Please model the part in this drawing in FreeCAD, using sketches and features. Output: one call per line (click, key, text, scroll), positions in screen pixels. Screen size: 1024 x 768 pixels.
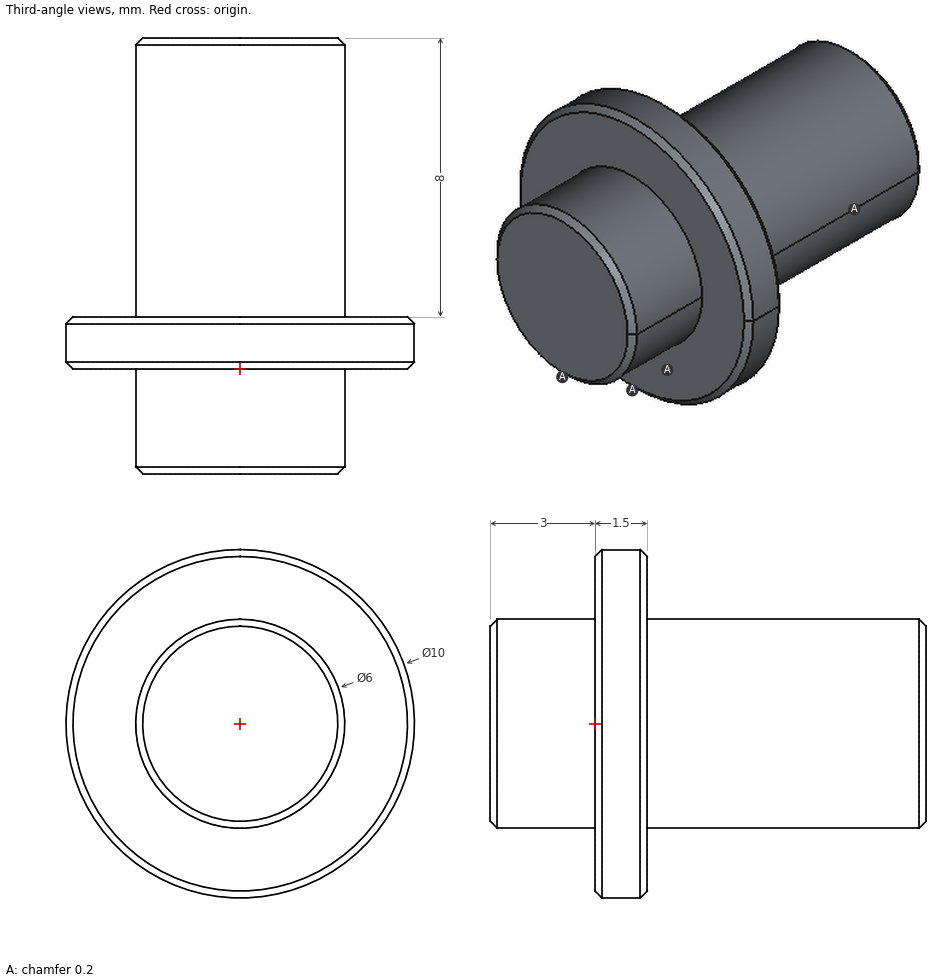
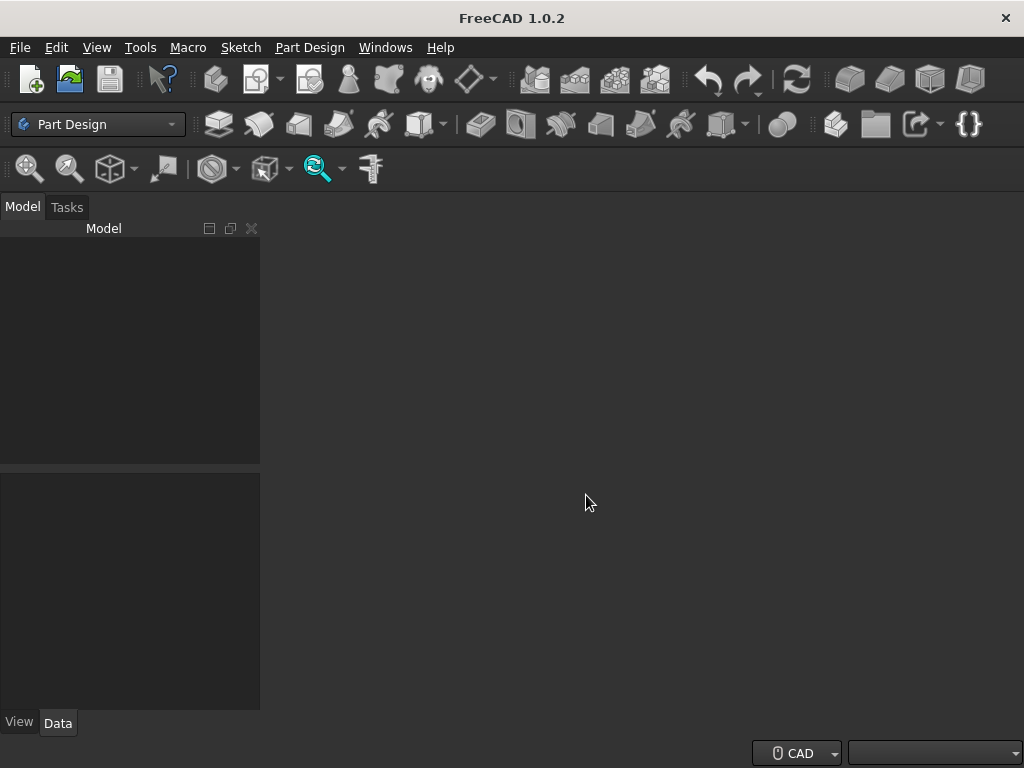
key(ctrl+n)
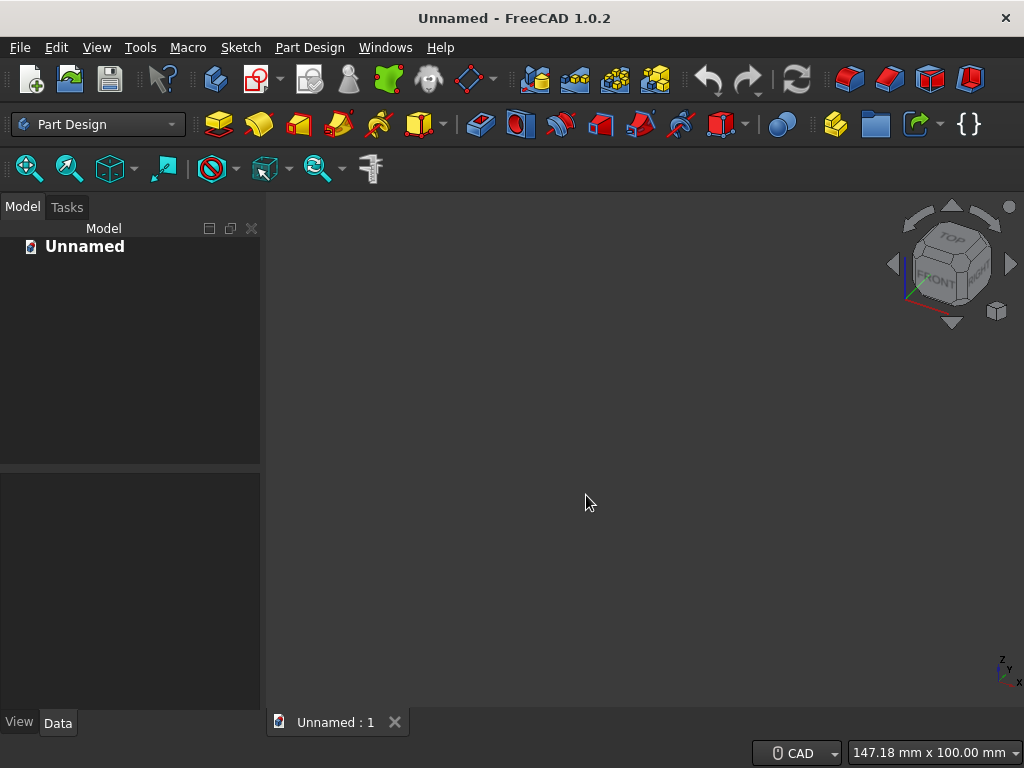
click(256, 80)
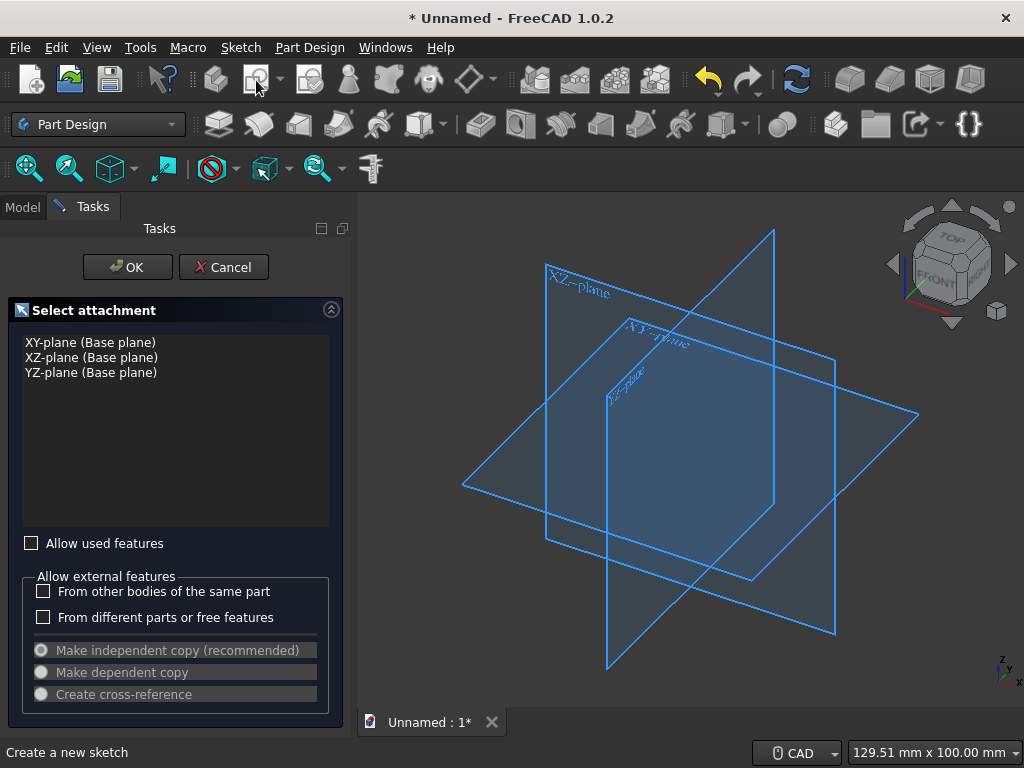
click(82, 358)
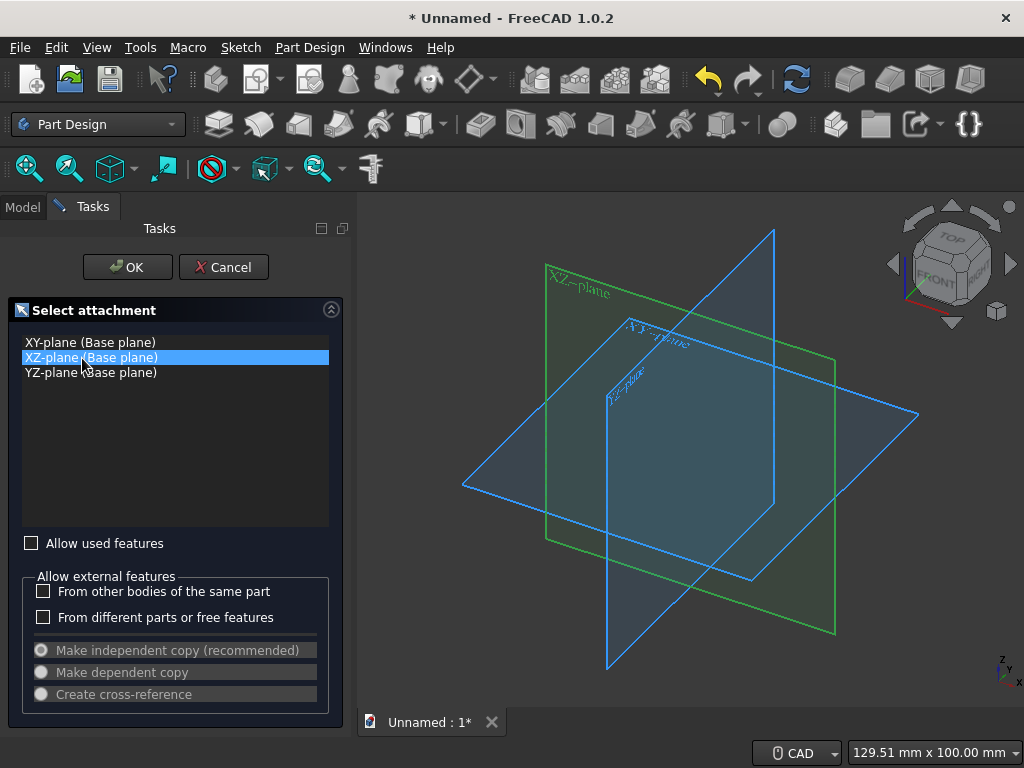
click(128, 267)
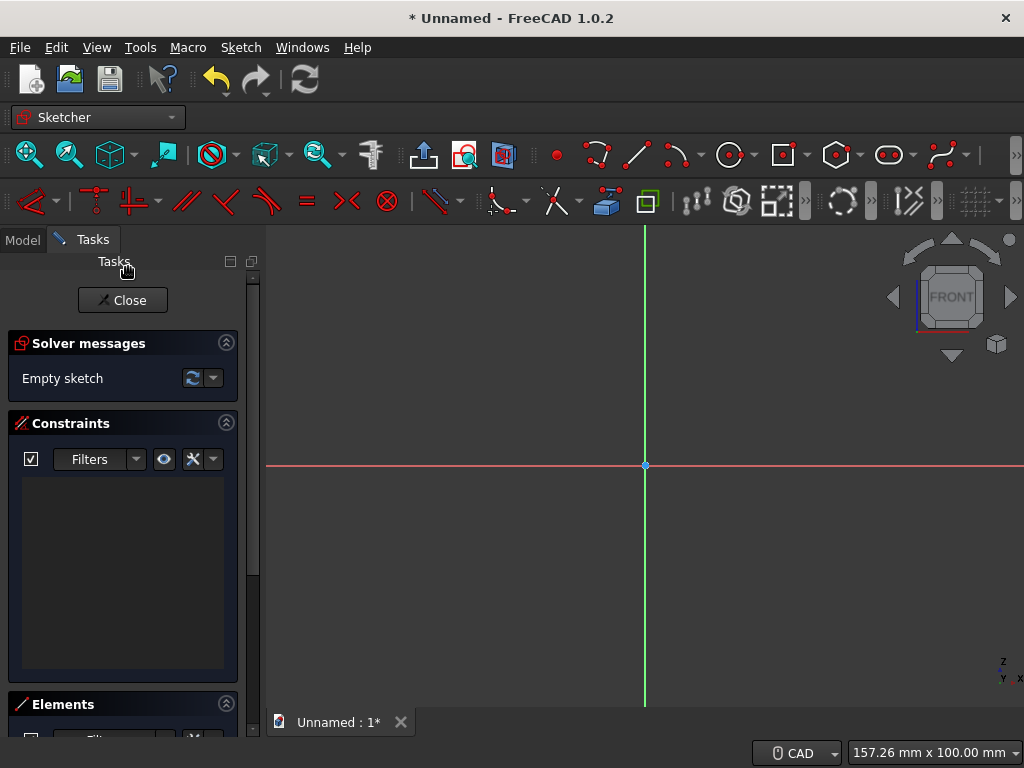
scroll(659, 466, up, 9)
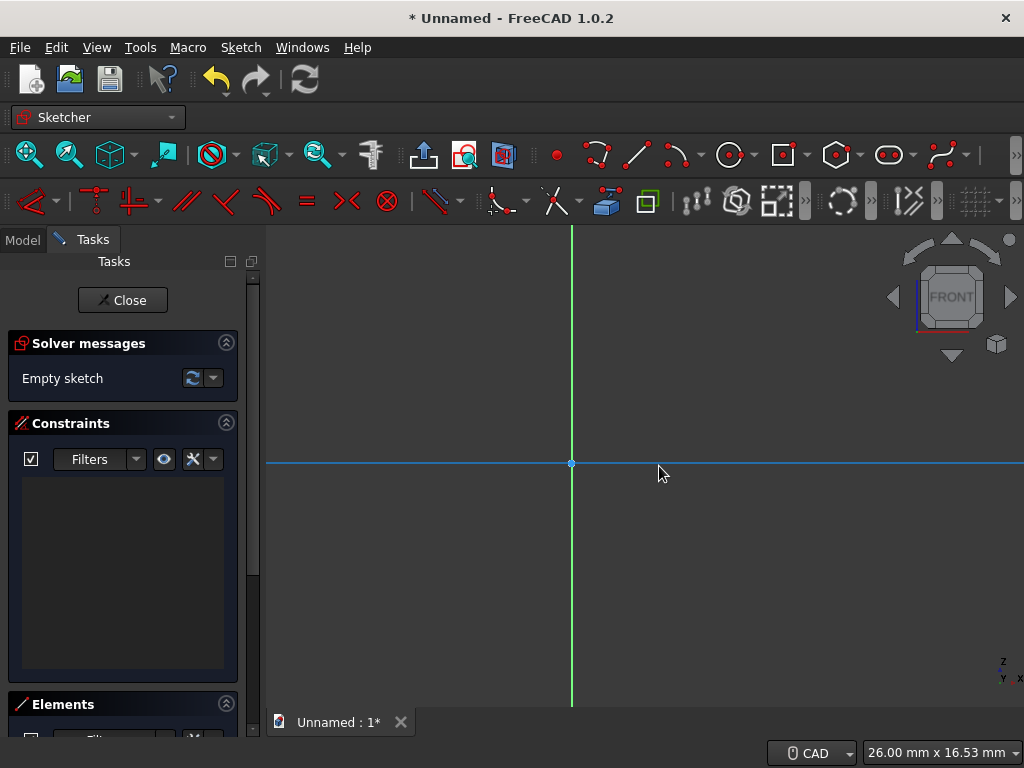
click(730, 156)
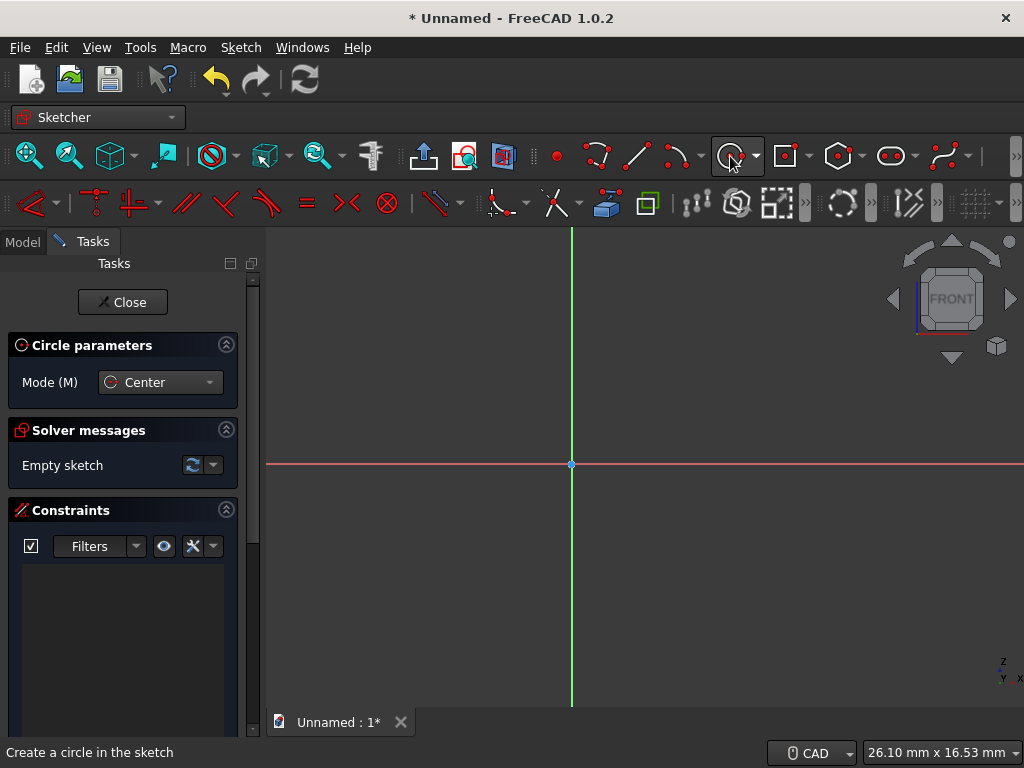
click(572, 464)
move(675, 362)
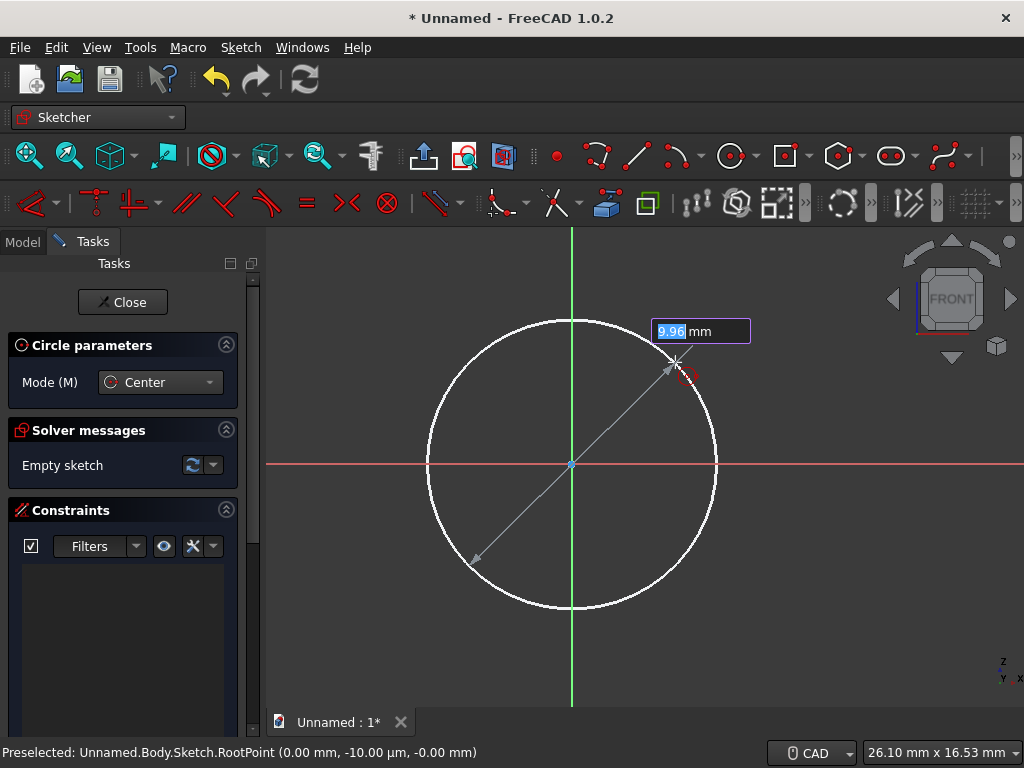
text(10)
key(Return)
key(Escape)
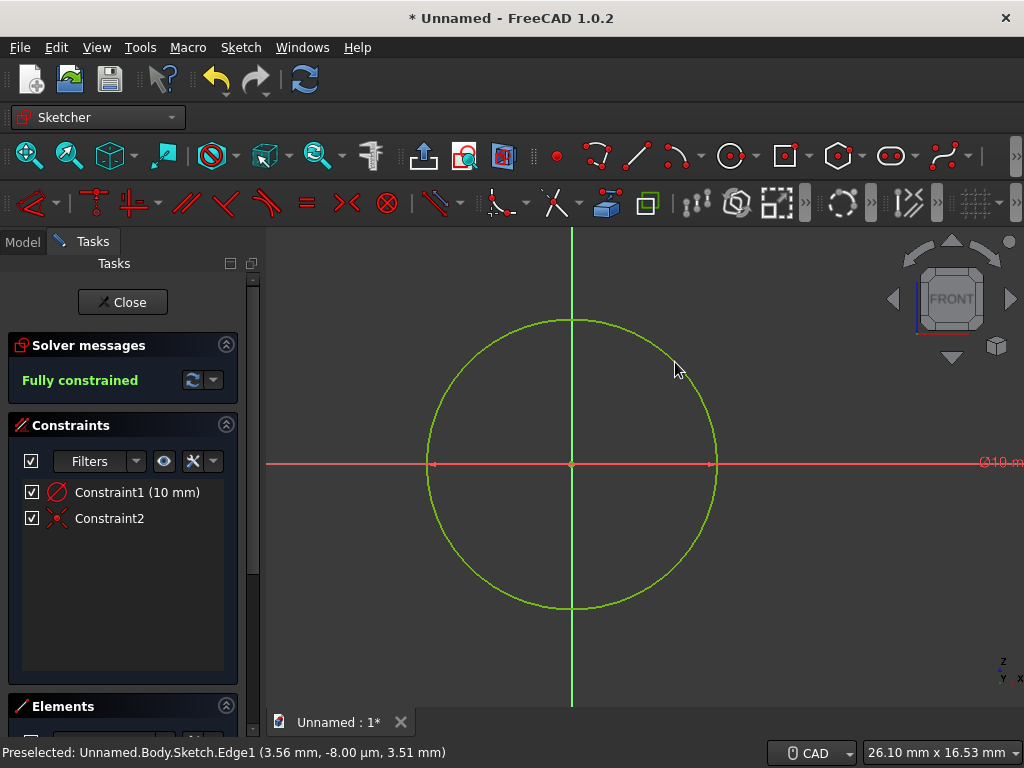
click(123, 302)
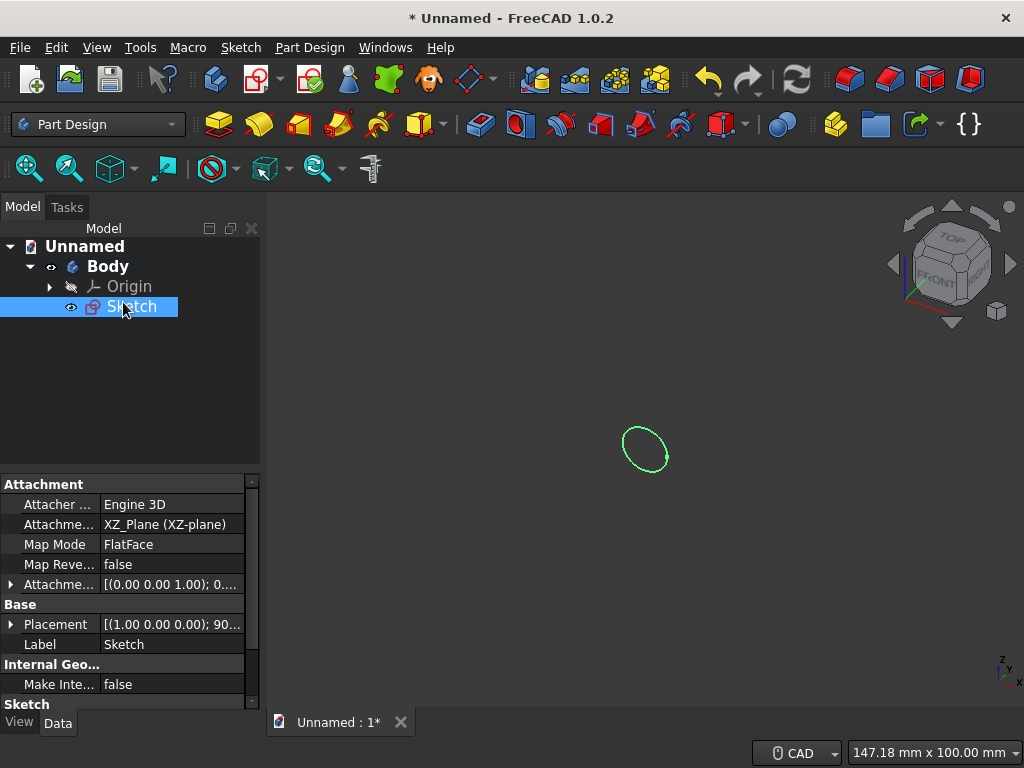
click(220, 124)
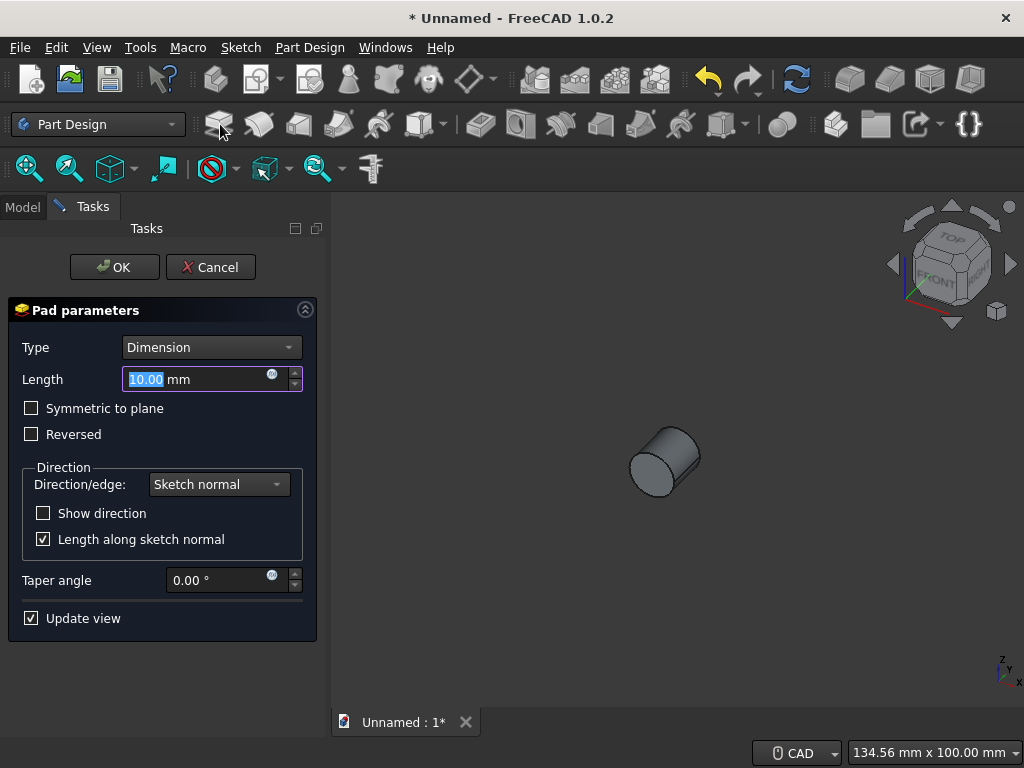
text(1.5)
key(Tab)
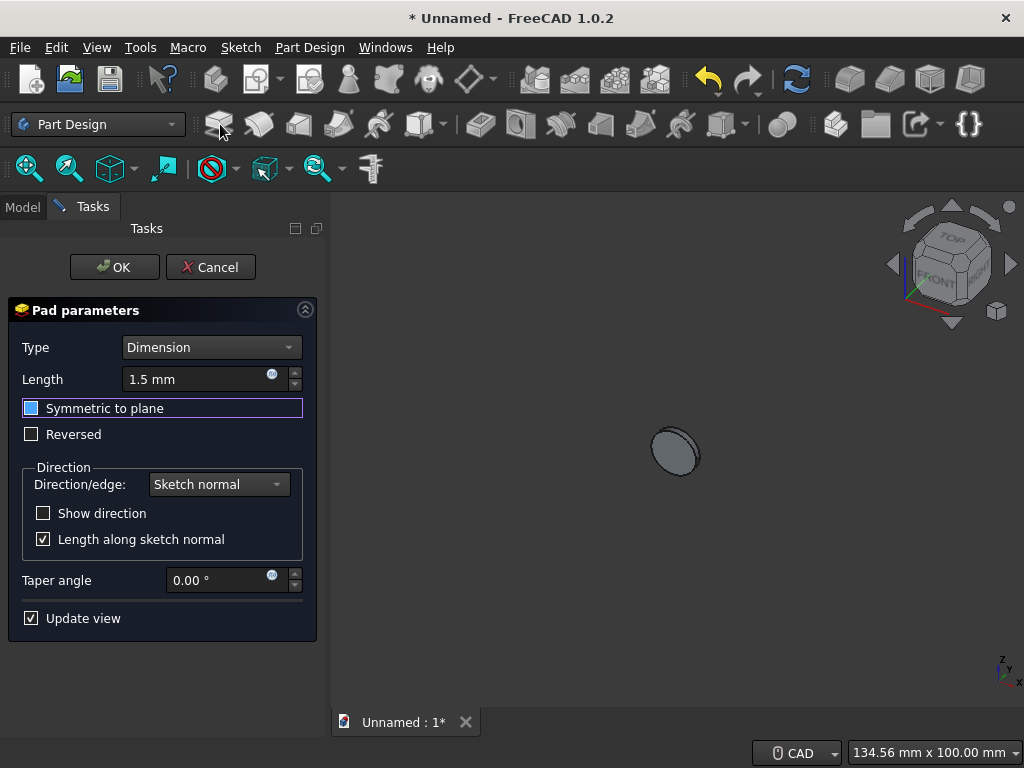
click(30, 434)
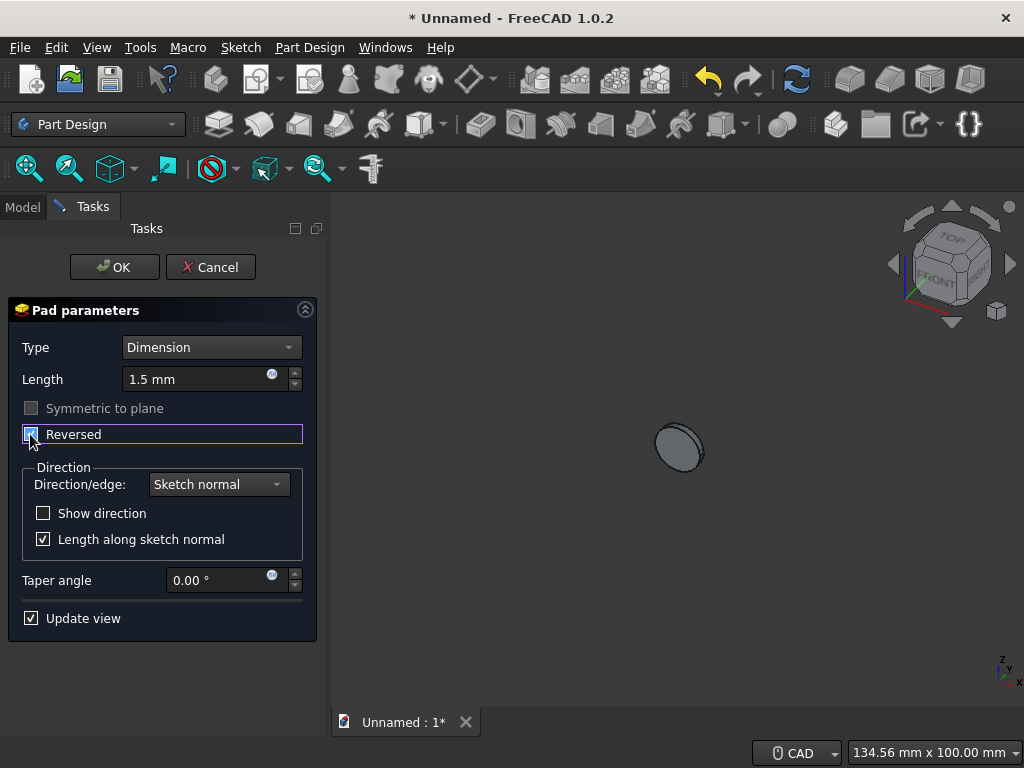
click(115, 267)